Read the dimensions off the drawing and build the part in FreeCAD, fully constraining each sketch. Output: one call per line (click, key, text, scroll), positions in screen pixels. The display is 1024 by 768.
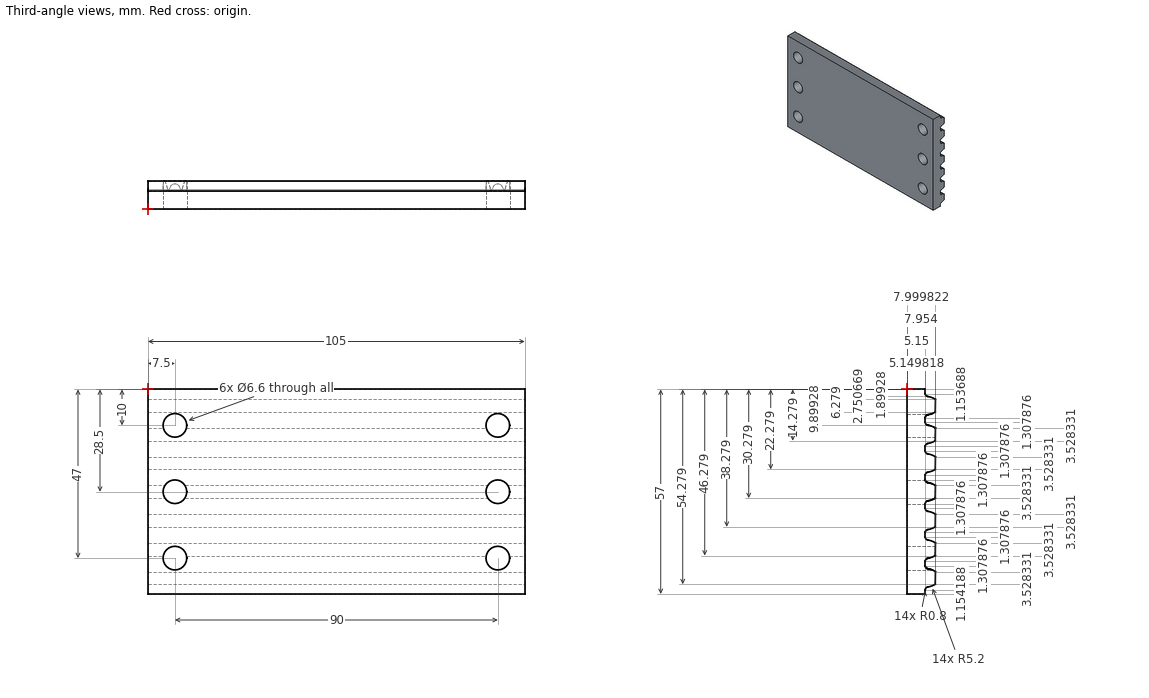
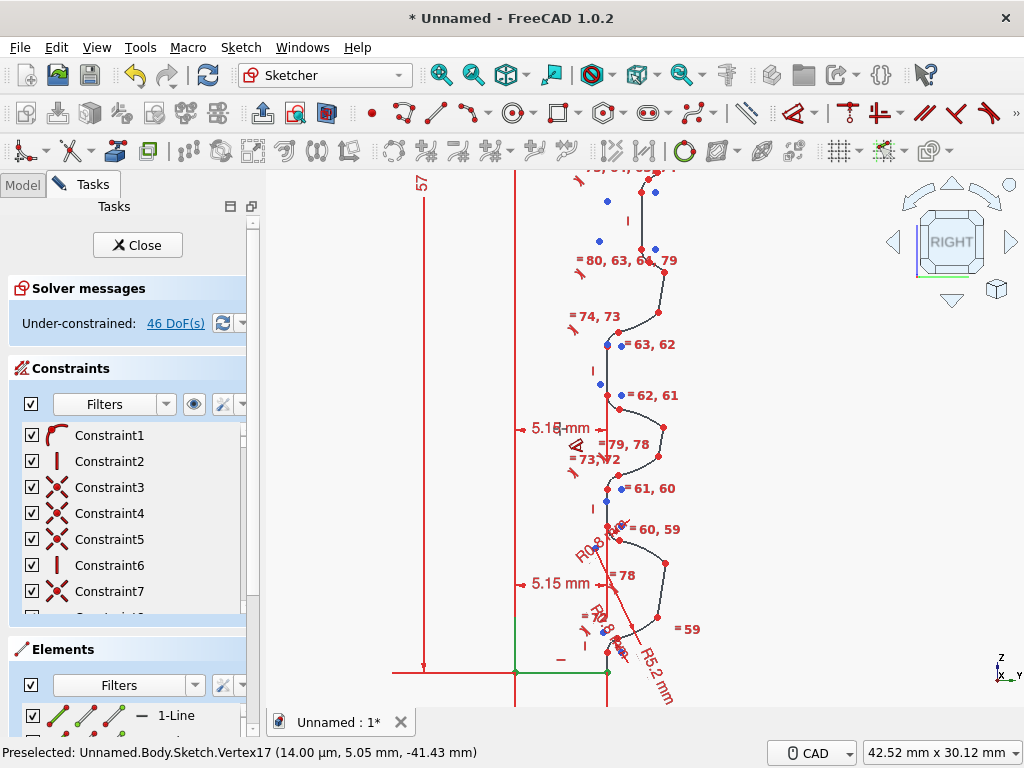
click(642, 249)
click(578, 283)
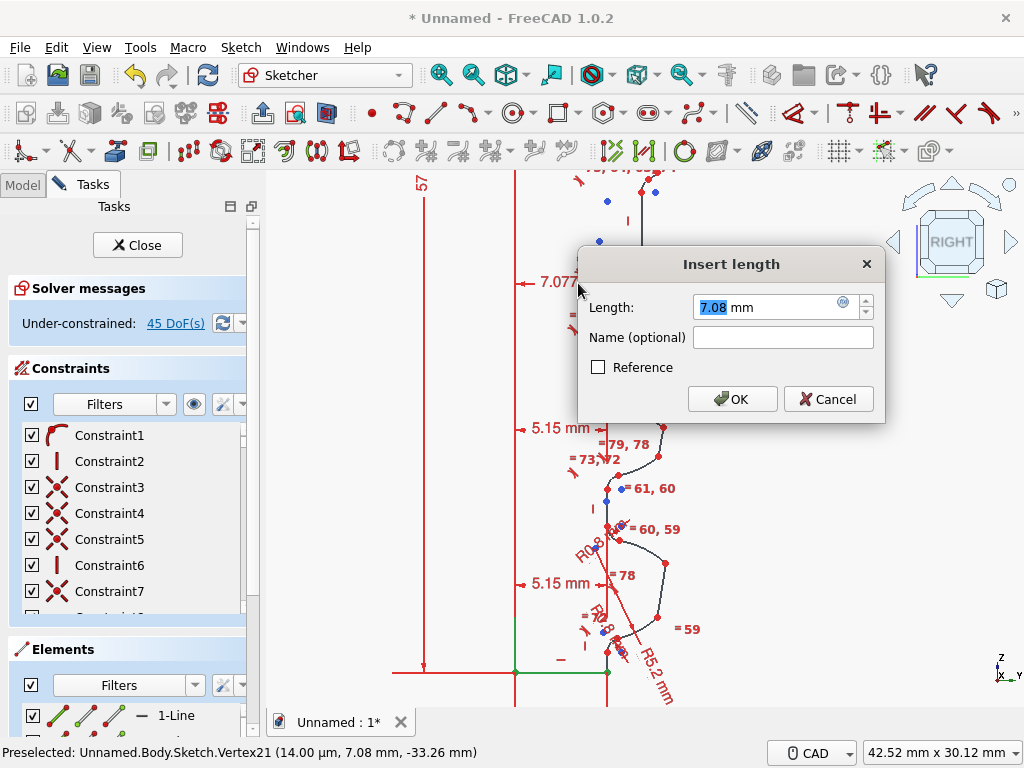
text(5.15)
key(Return)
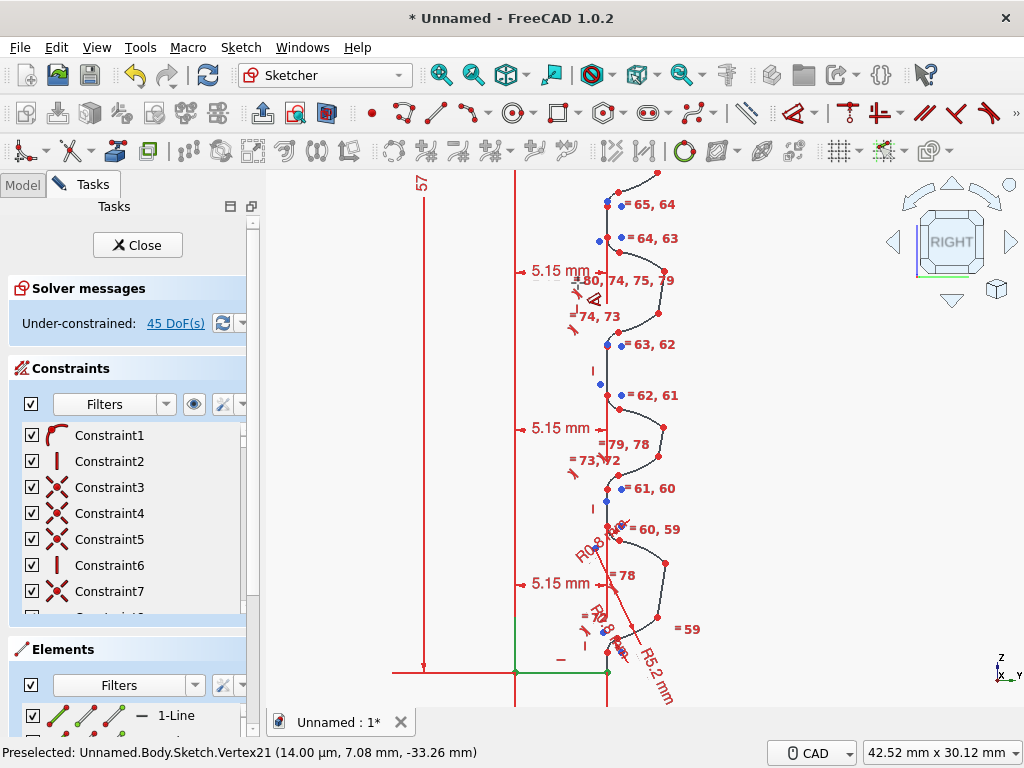
scroll(571, 598, down, 5)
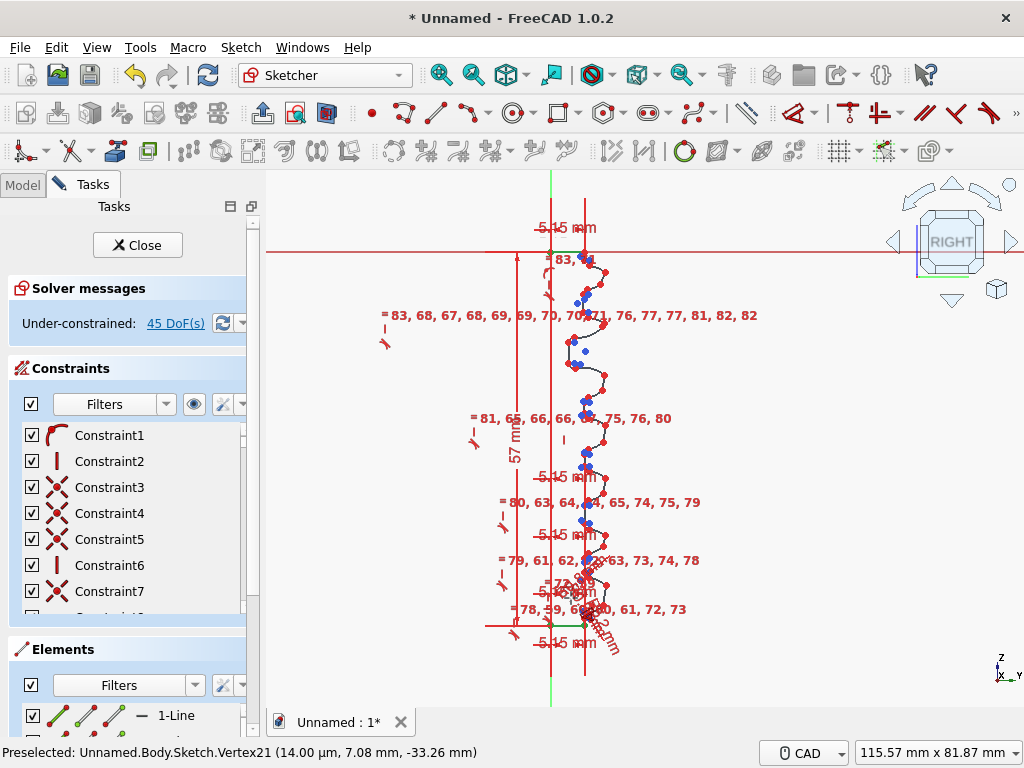
scroll(584, 413, up, 6)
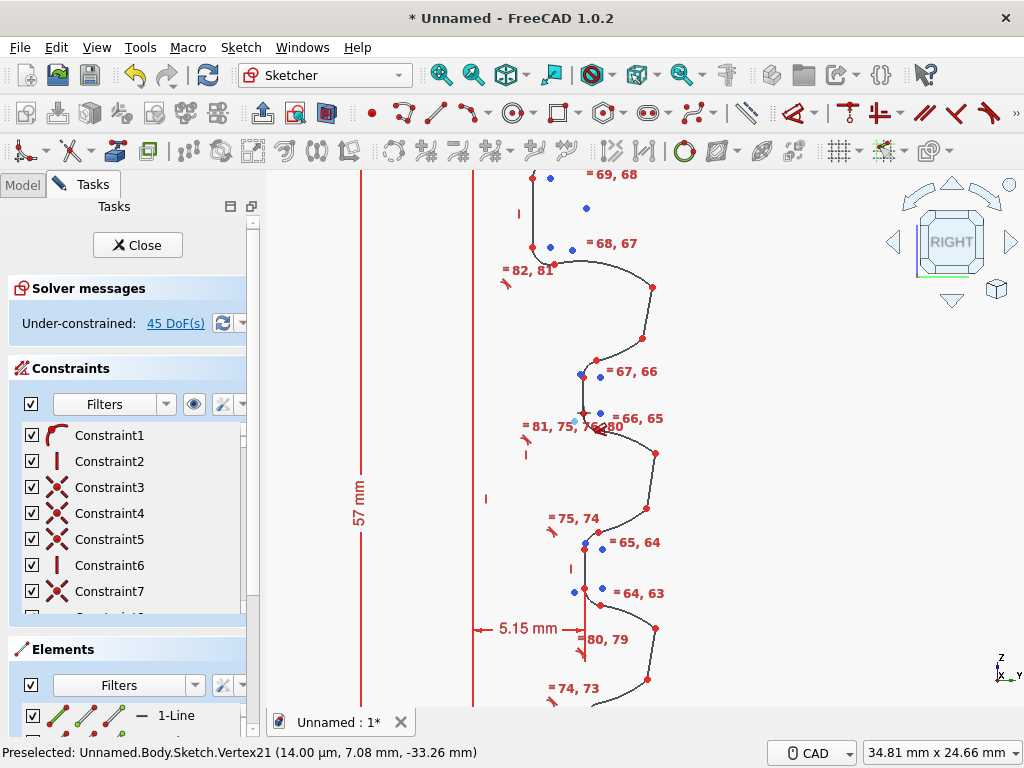
click(583, 413)
click(528, 447)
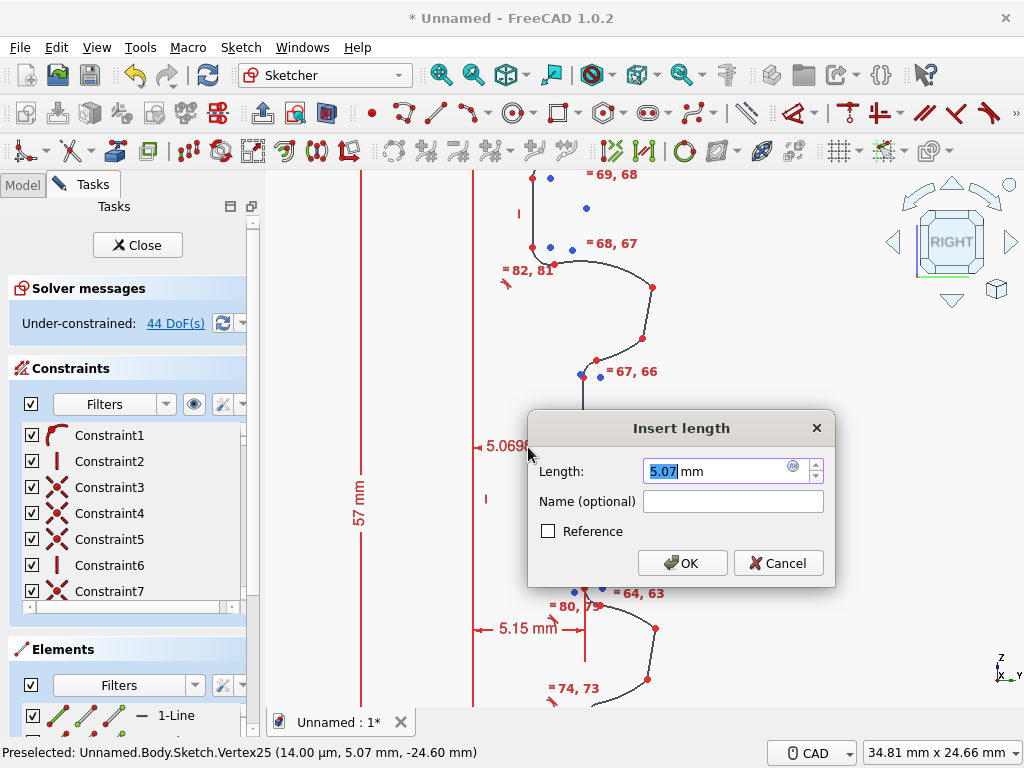
text(5.15)
key(Return)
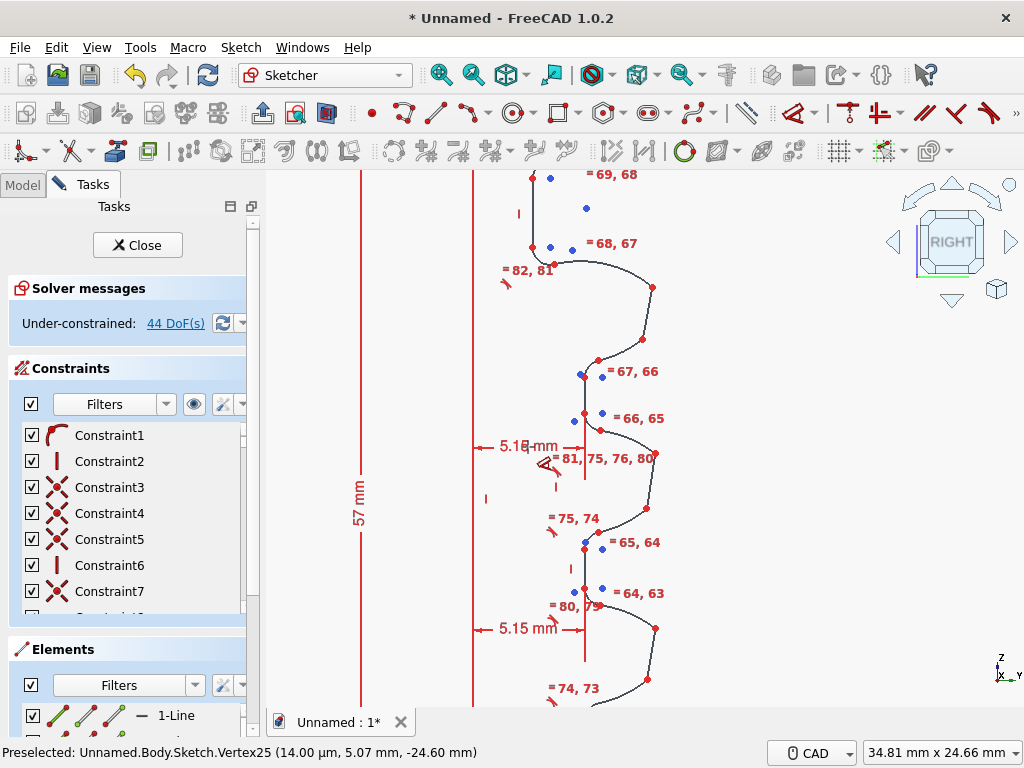
click(533, 247)
click(503, 281)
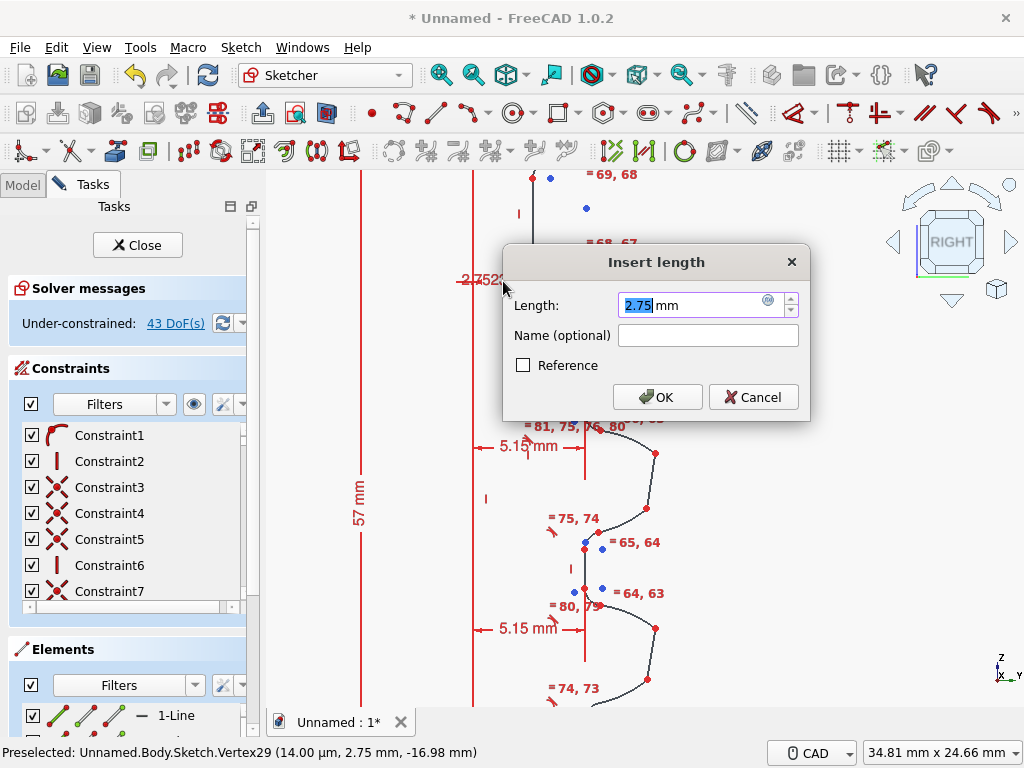
text(5.15)
key(Return)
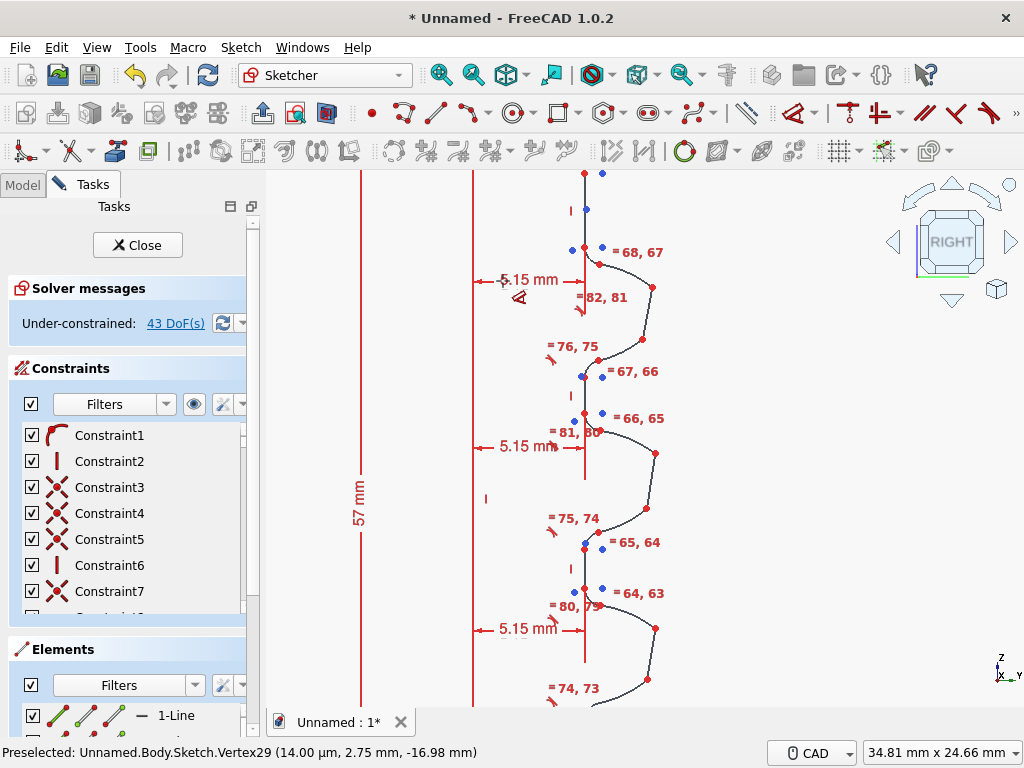
scroll(584, 413, down, 6)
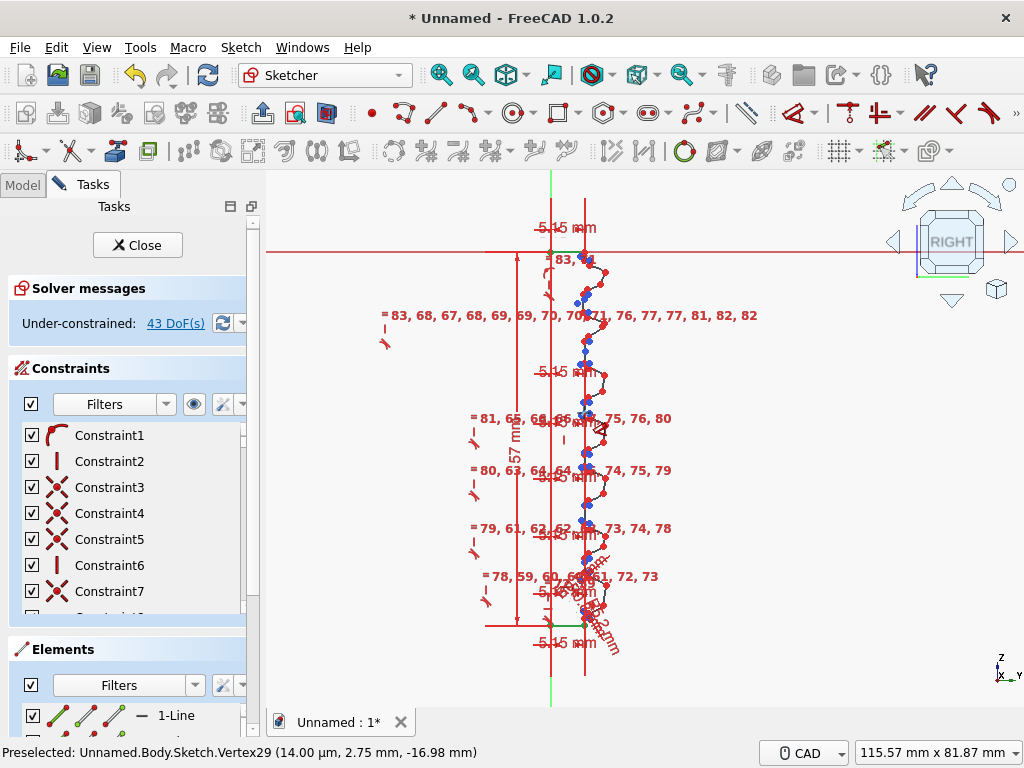
scroll(583, 313, up, 5)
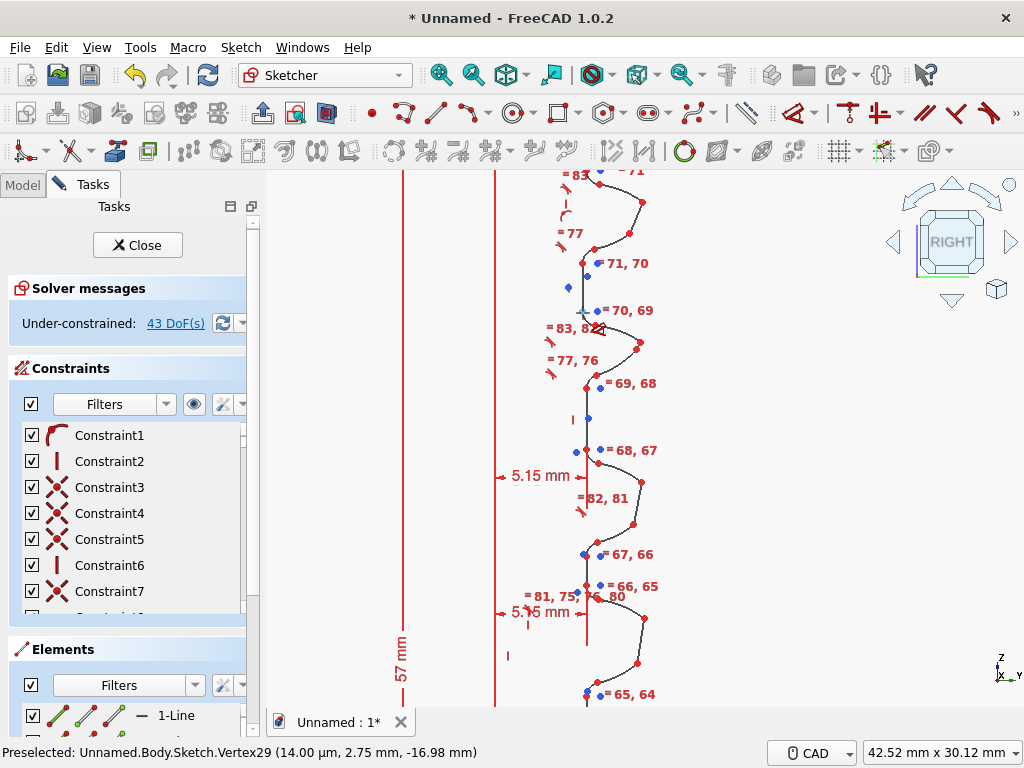
click(583, 312)
click(539, 346)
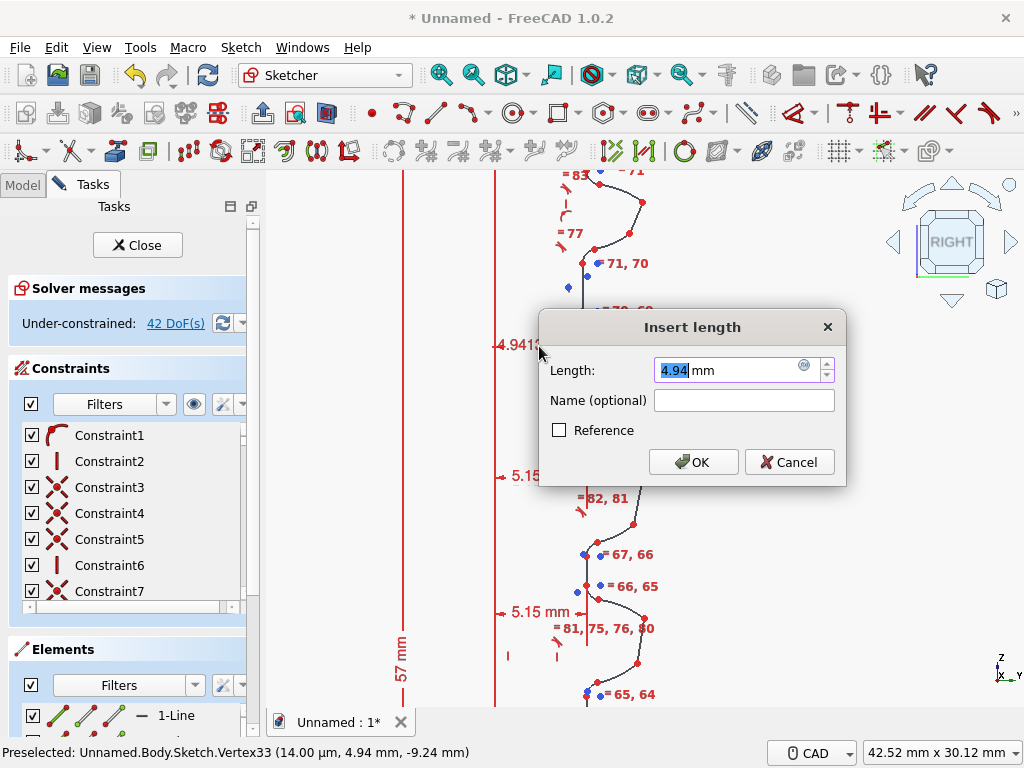
text(5.15)
key(Return)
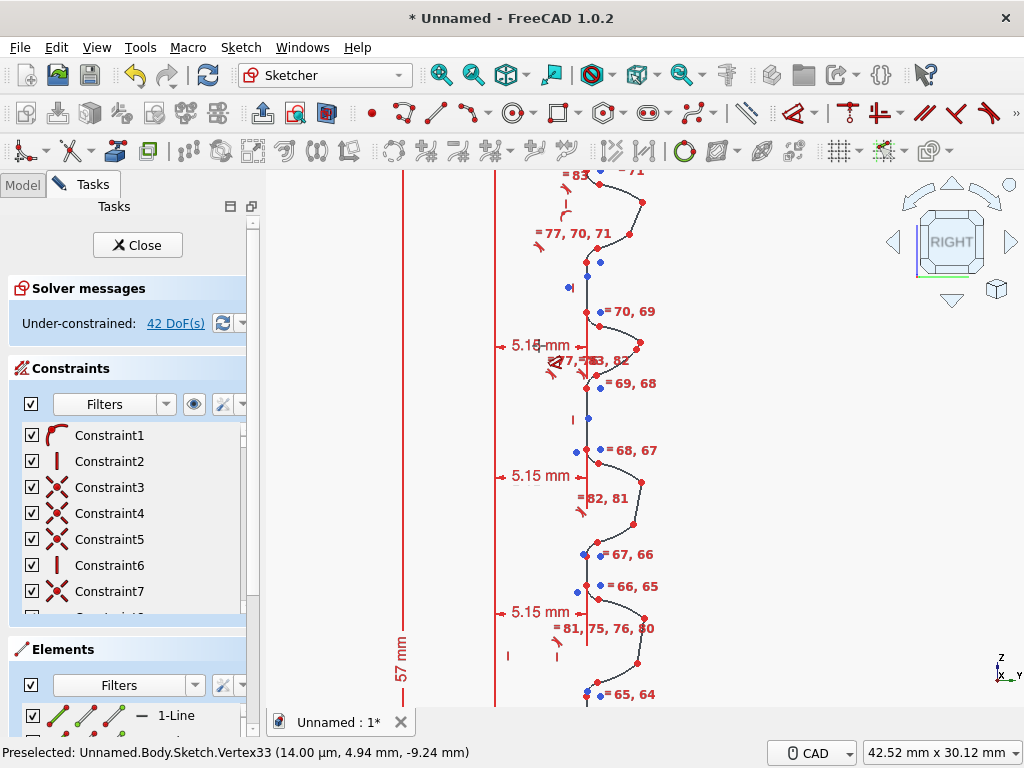
scroll(583, 312, down, 5)